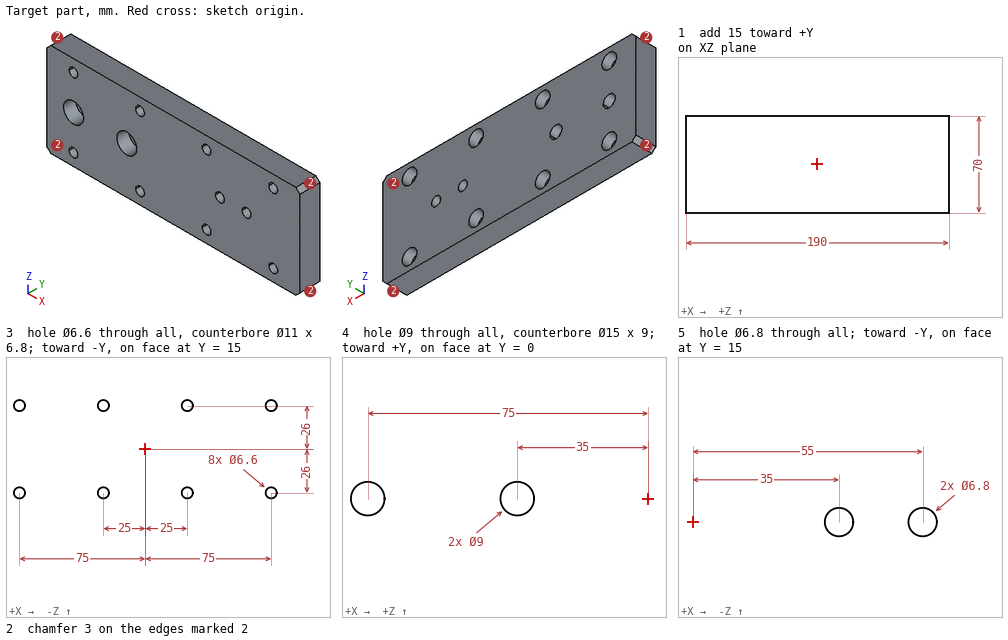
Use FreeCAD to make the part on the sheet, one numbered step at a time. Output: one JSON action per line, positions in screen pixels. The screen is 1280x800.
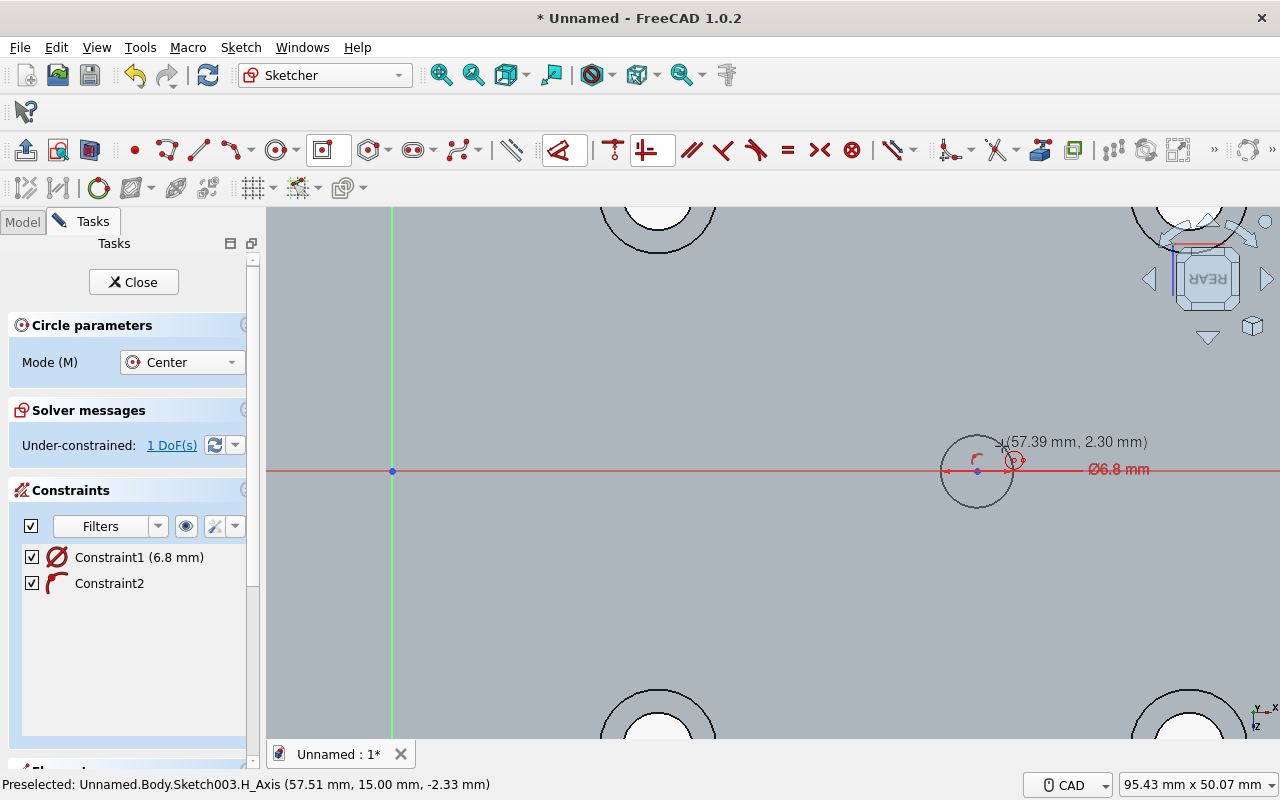
{"action": "left_click", "coordinate": [764, 471]}
{"action": "mouse_move", "coordinate": [790, 446]}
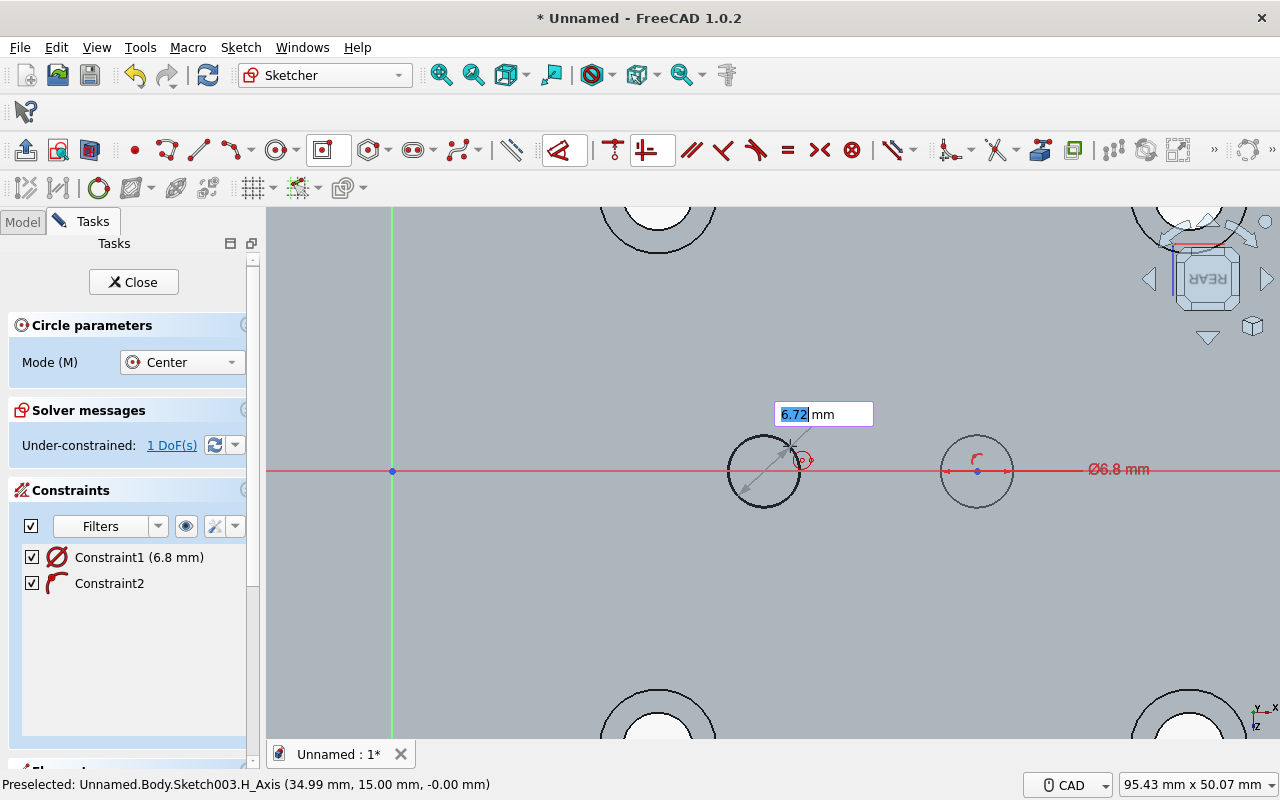
{"action": "type", "text": "6.8"}
{"action": "key", "text": "Return"}
{"action": "key", "text": "Escape"}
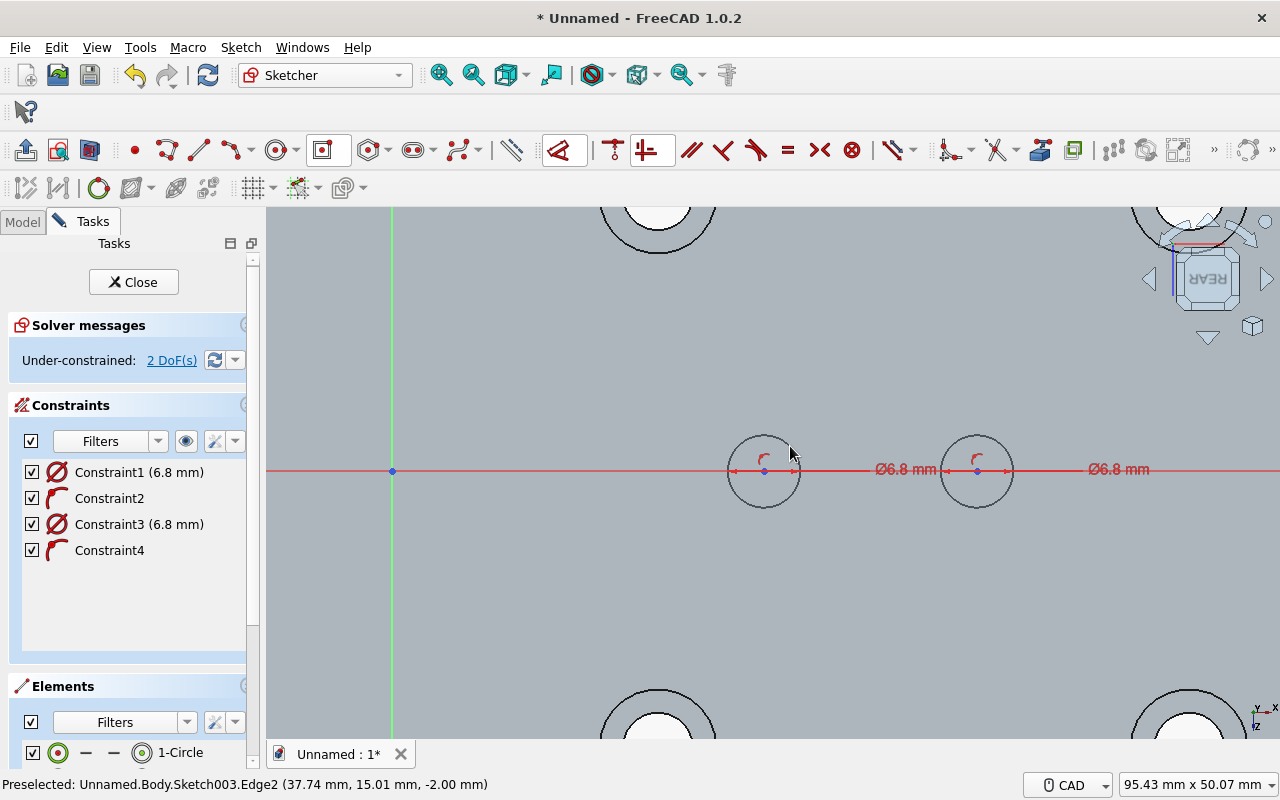
{"action": "key", "text": "d"}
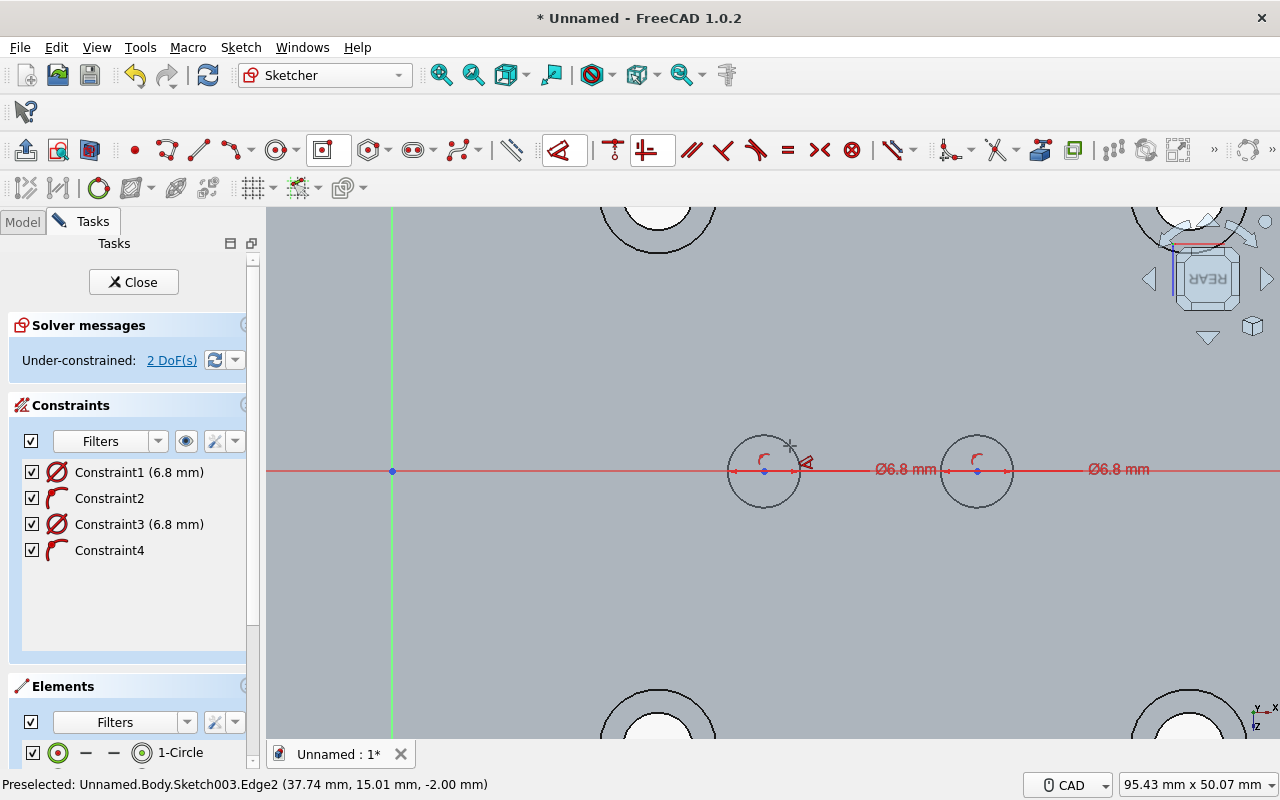
{"action": "left_click", "coordinate": [977, 471]}
{"action": "left_click", "coordinate": [685, 505]}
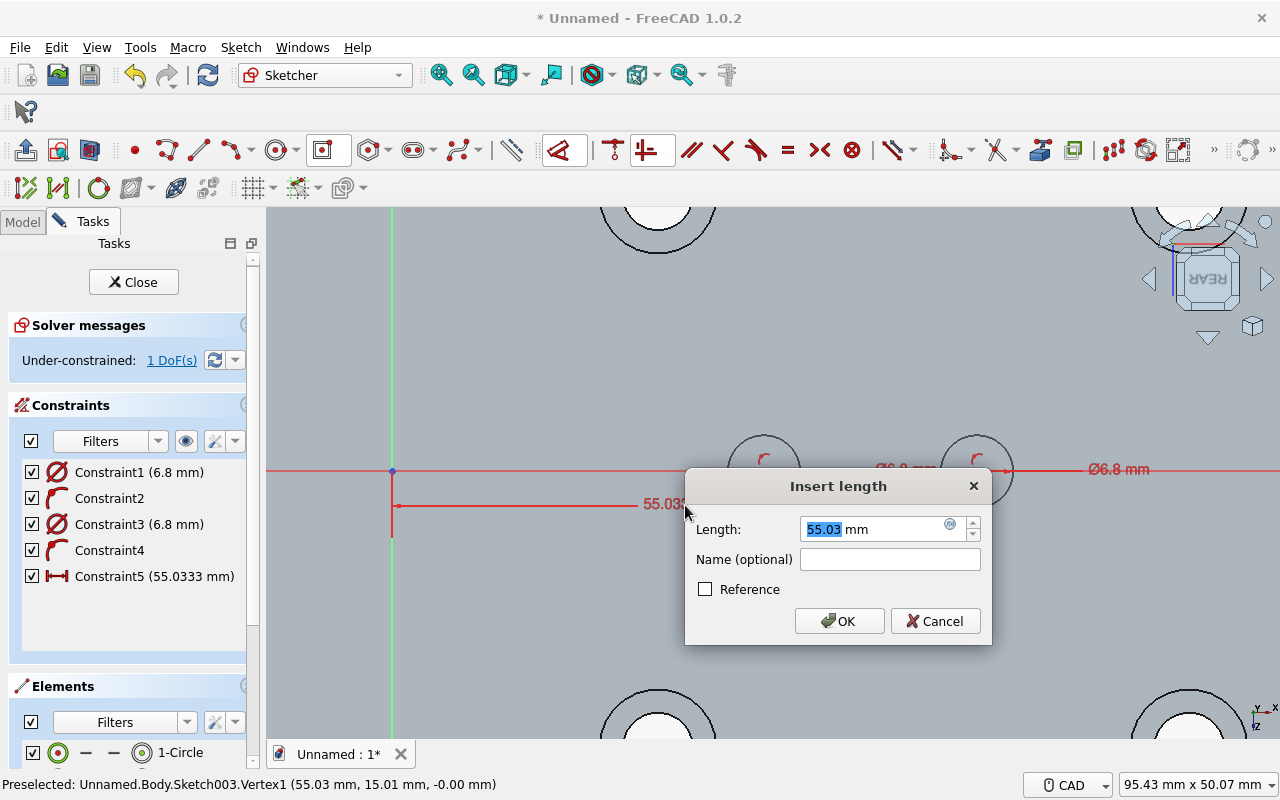
{"action": "type", "text": "55"}
{"action": "key", "text": "Return"}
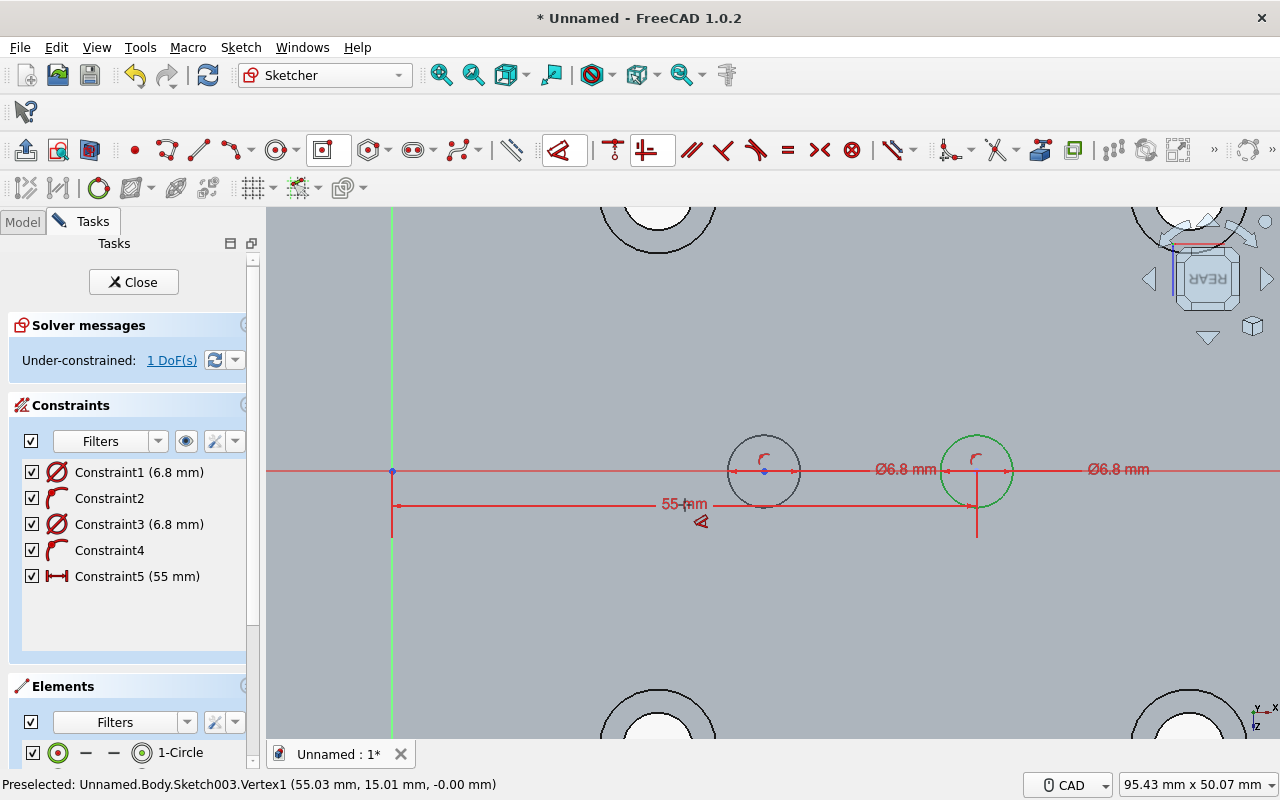
{"action": "left_click", "coordinate": [764, 471]}
{"action": "left_click", "coordinate": [578, 505]}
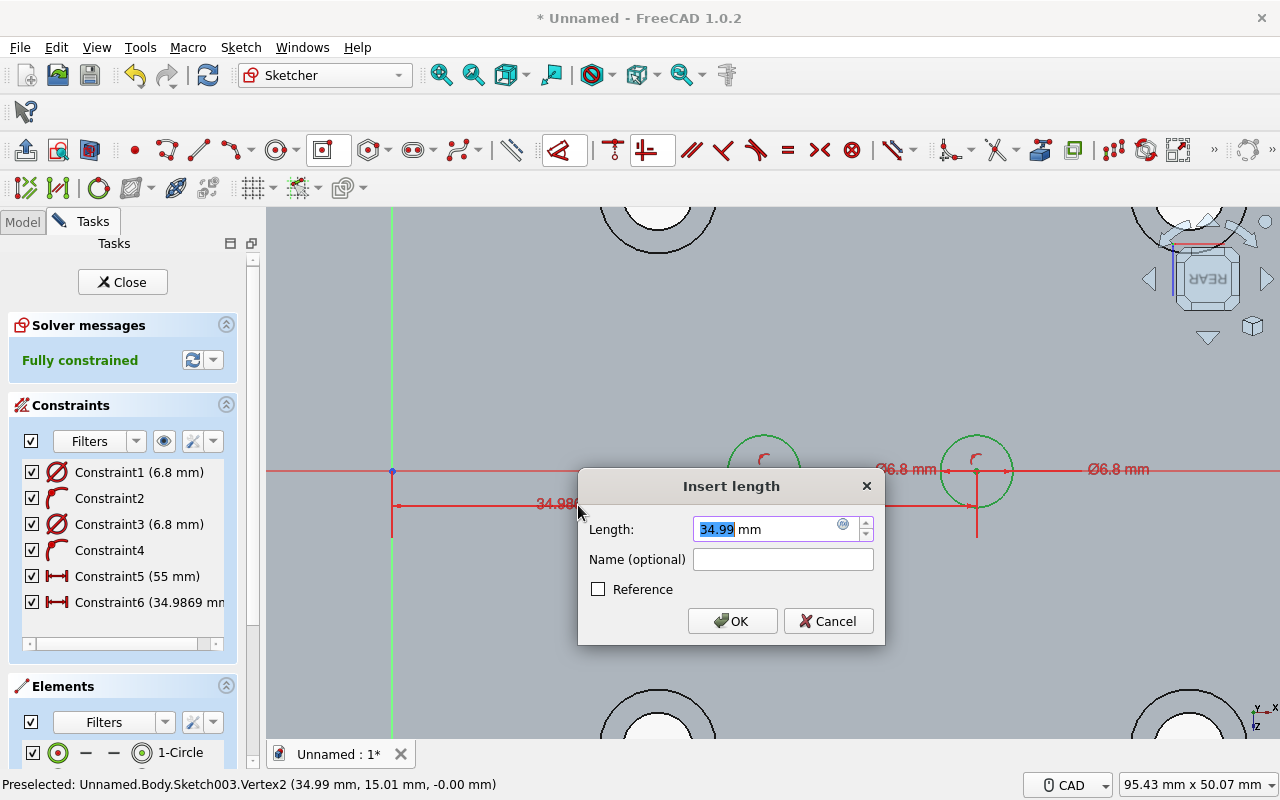
{"action": "type", "text": "35"}
{"action": "key", "text": "Return"}
{"action": "key", "text": "Escape"}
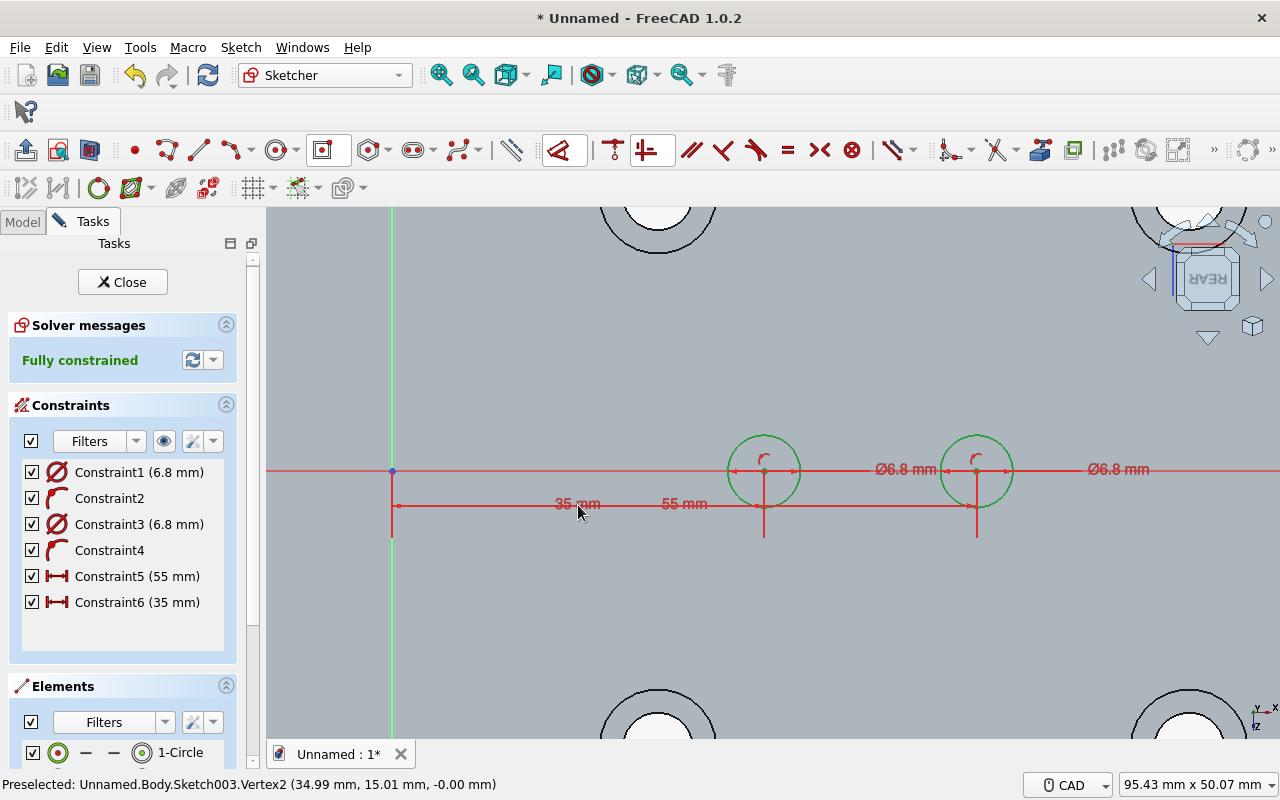
{"action": "left_click", "coordinate": [123, 282]}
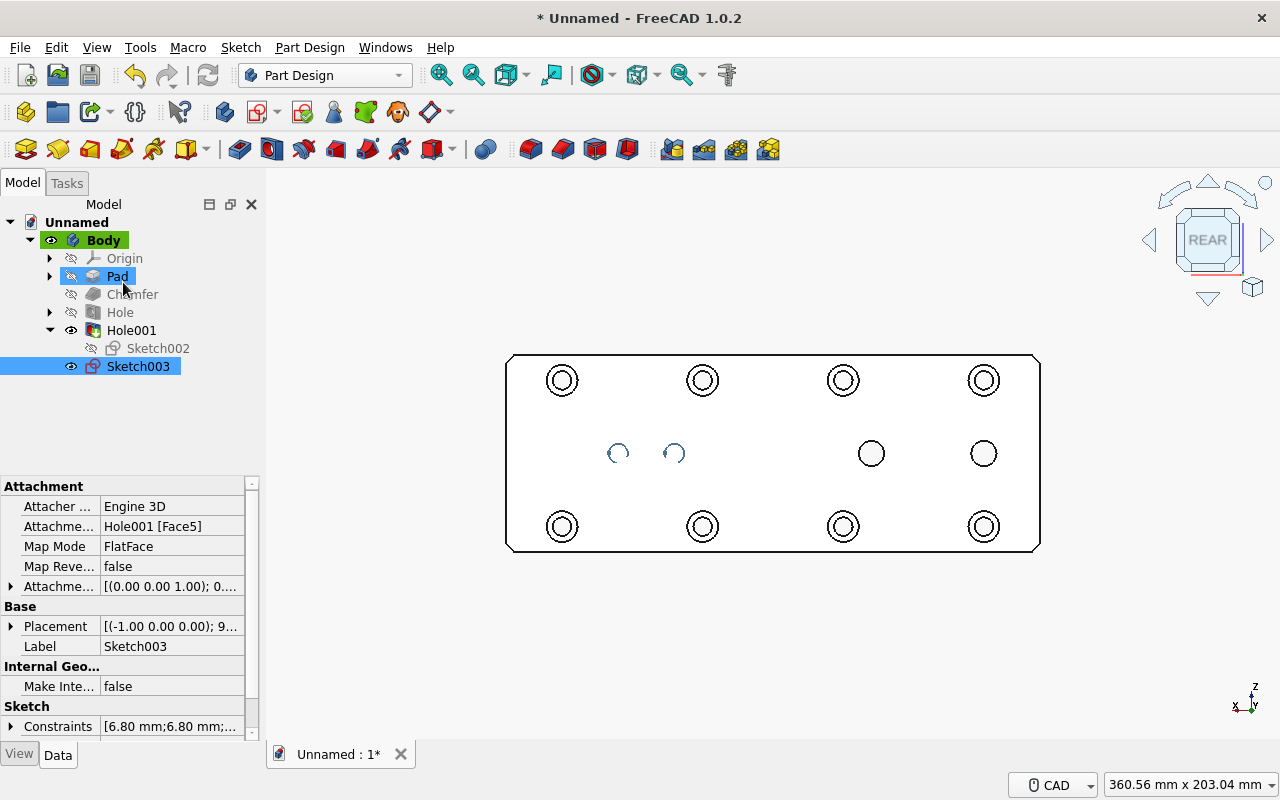
{"action": "left_click", "coordinate": [272, 150]}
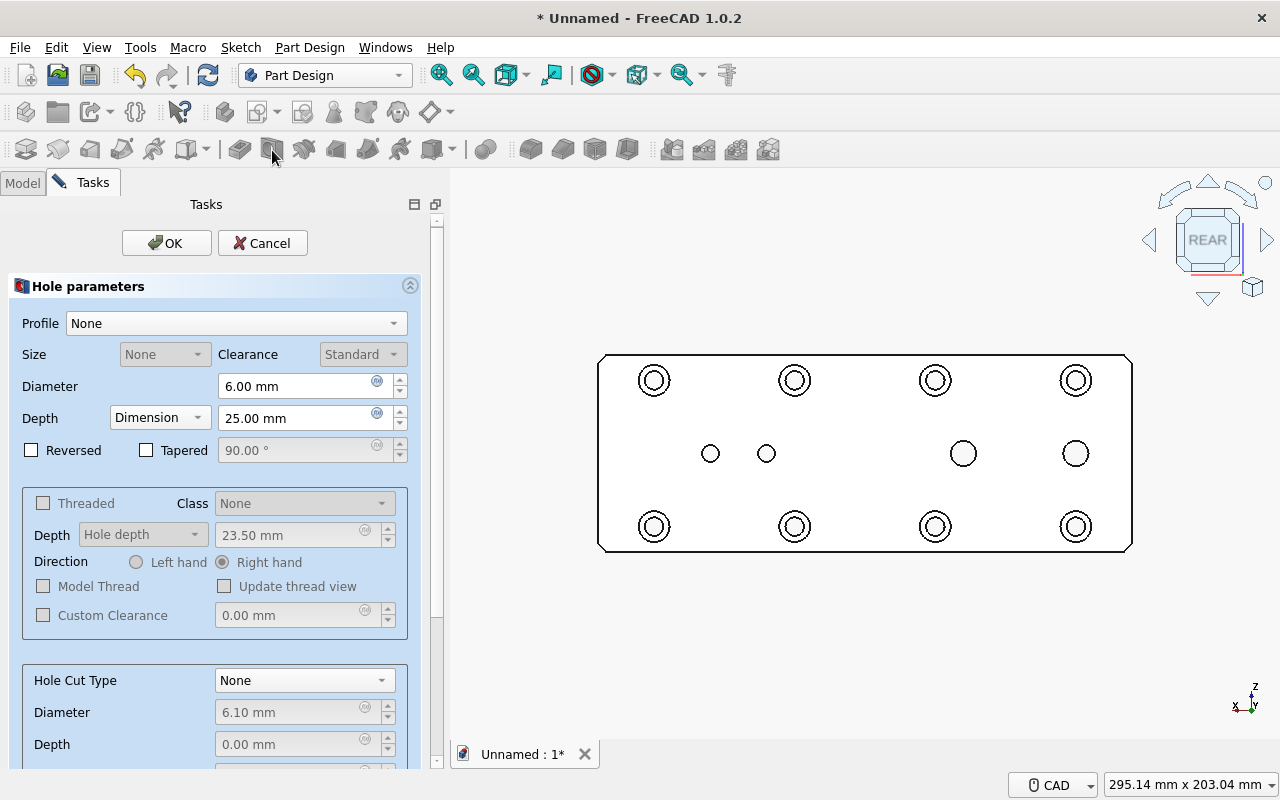
{"action": "triple_click", "coordinate": [305, 386]}